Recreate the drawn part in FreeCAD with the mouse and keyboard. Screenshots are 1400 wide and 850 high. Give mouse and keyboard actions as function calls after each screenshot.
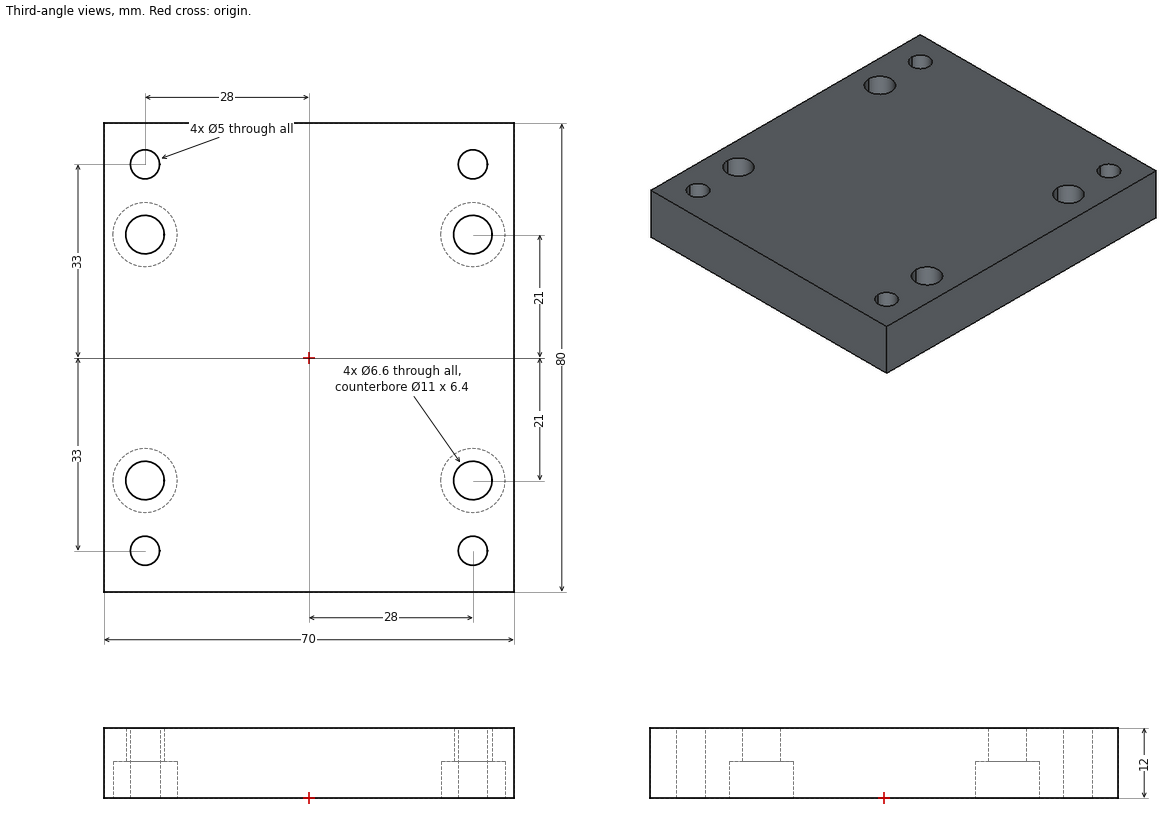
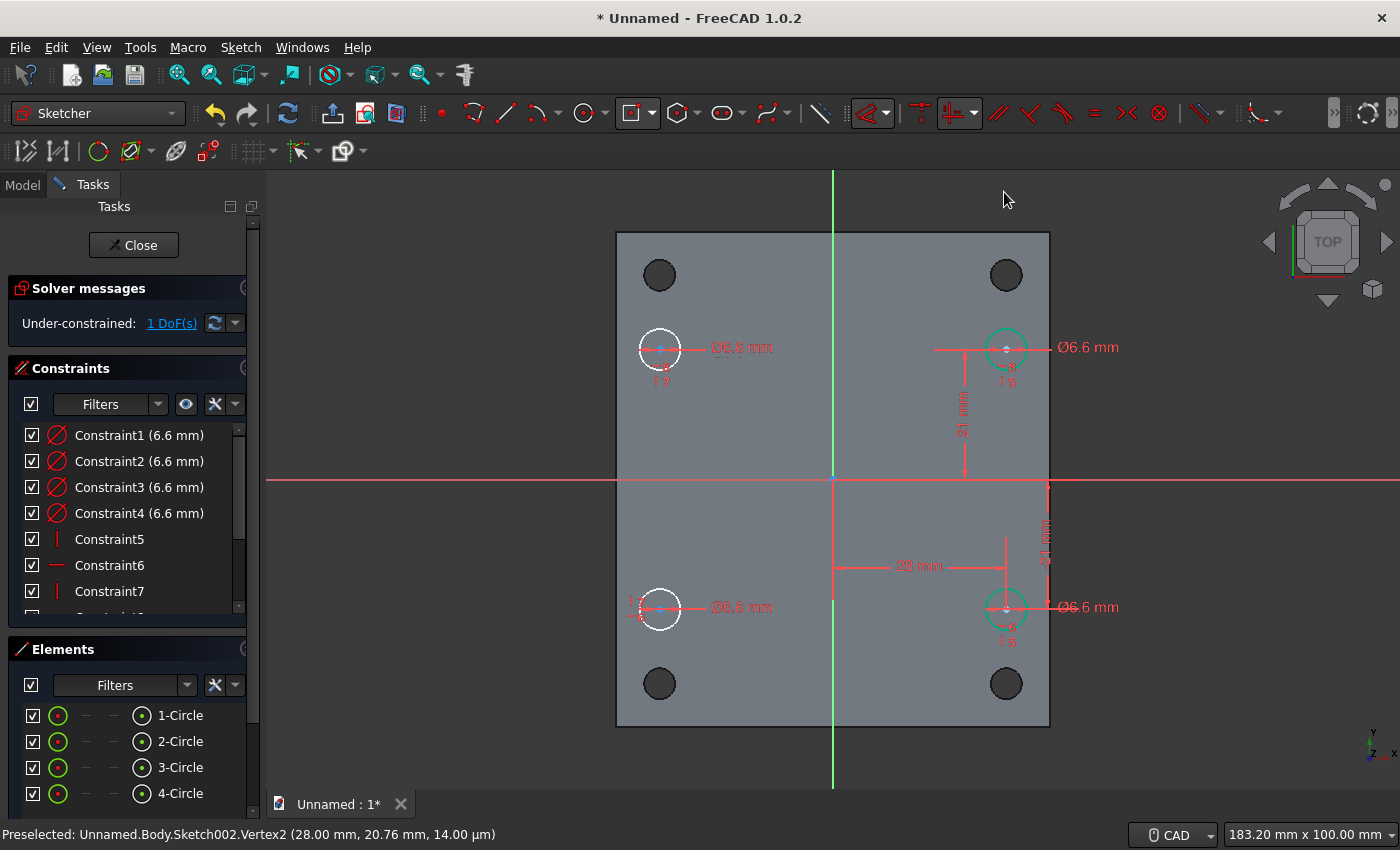
click(660, 609)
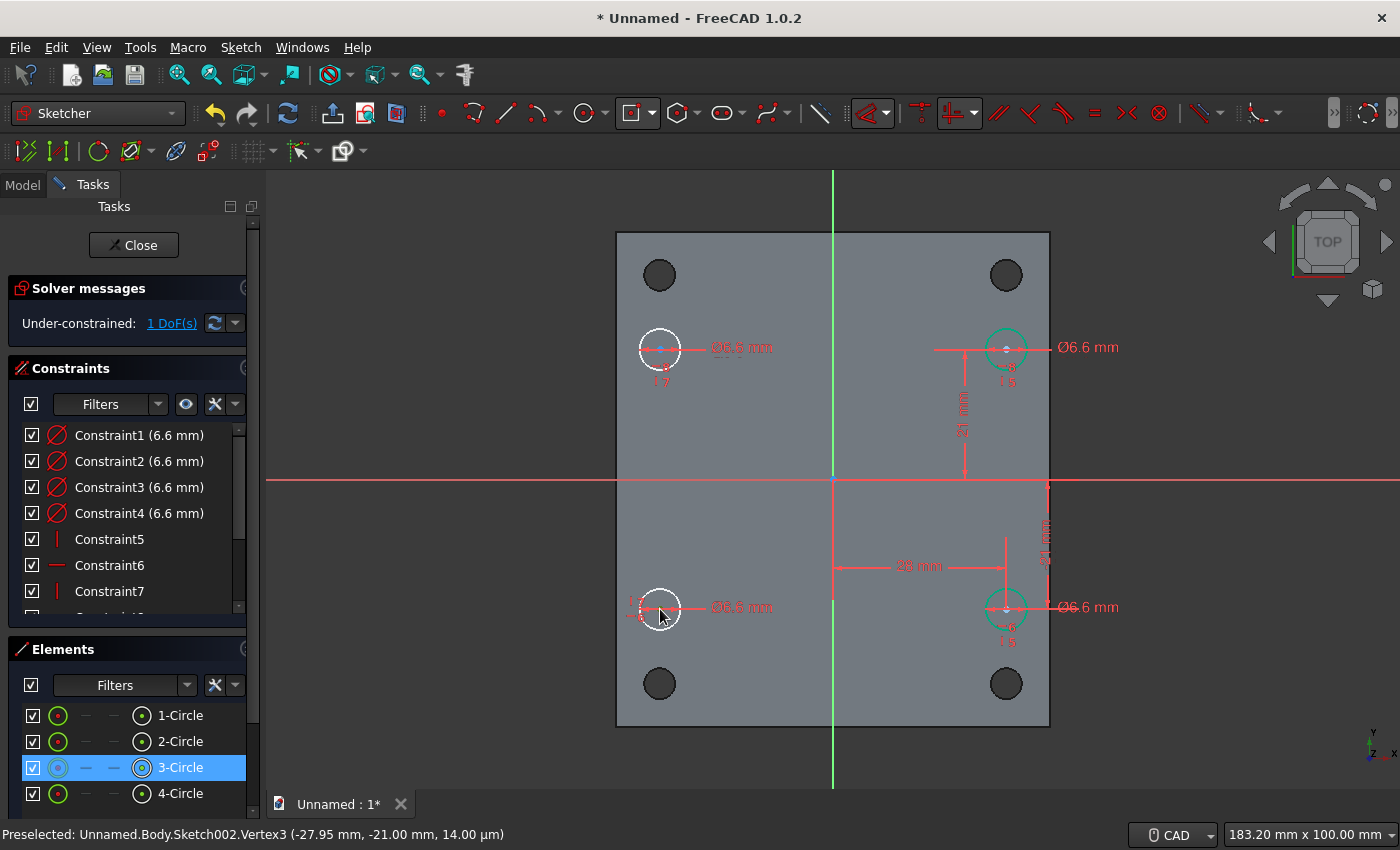
key(l)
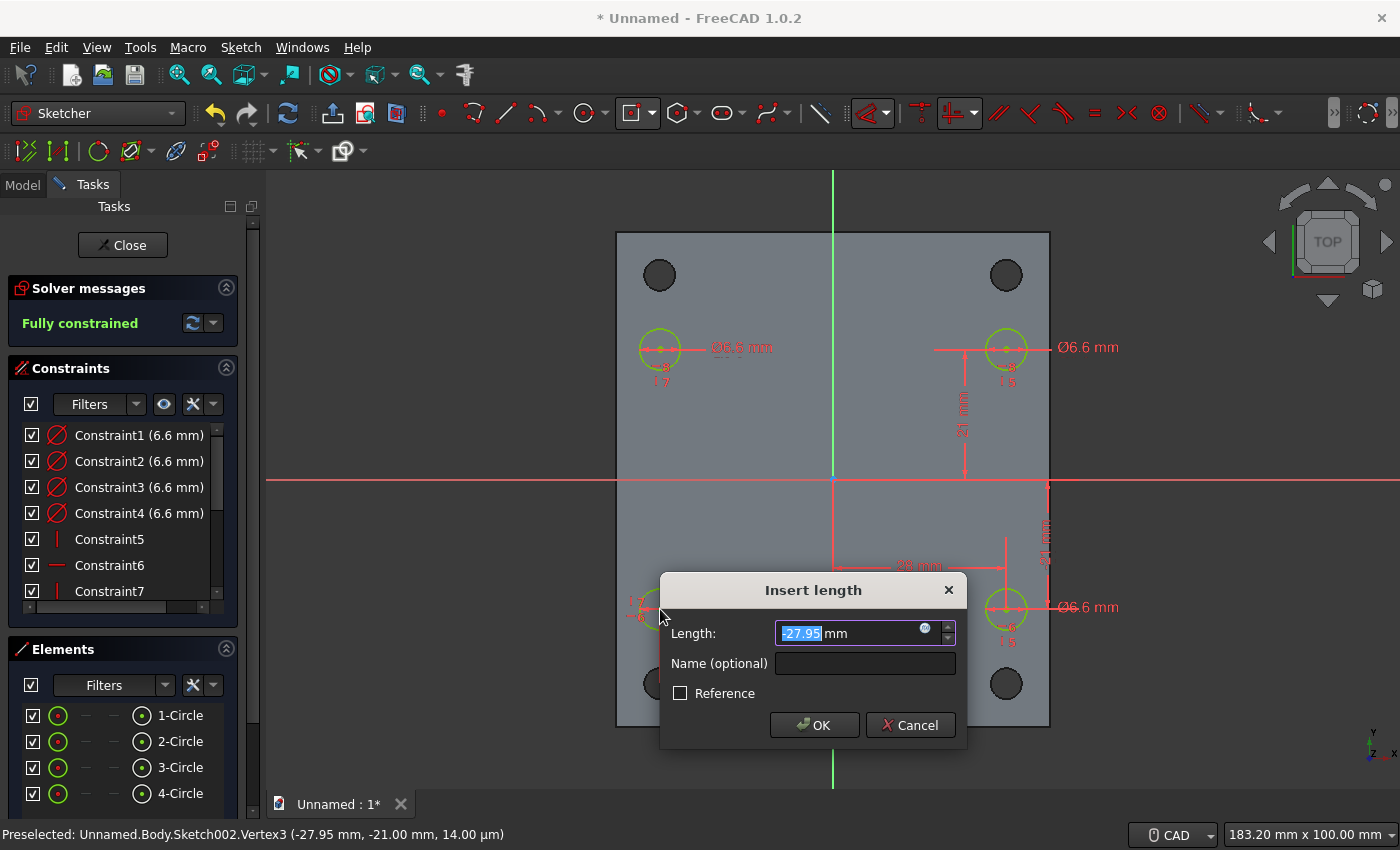
text(-28)
key(Return)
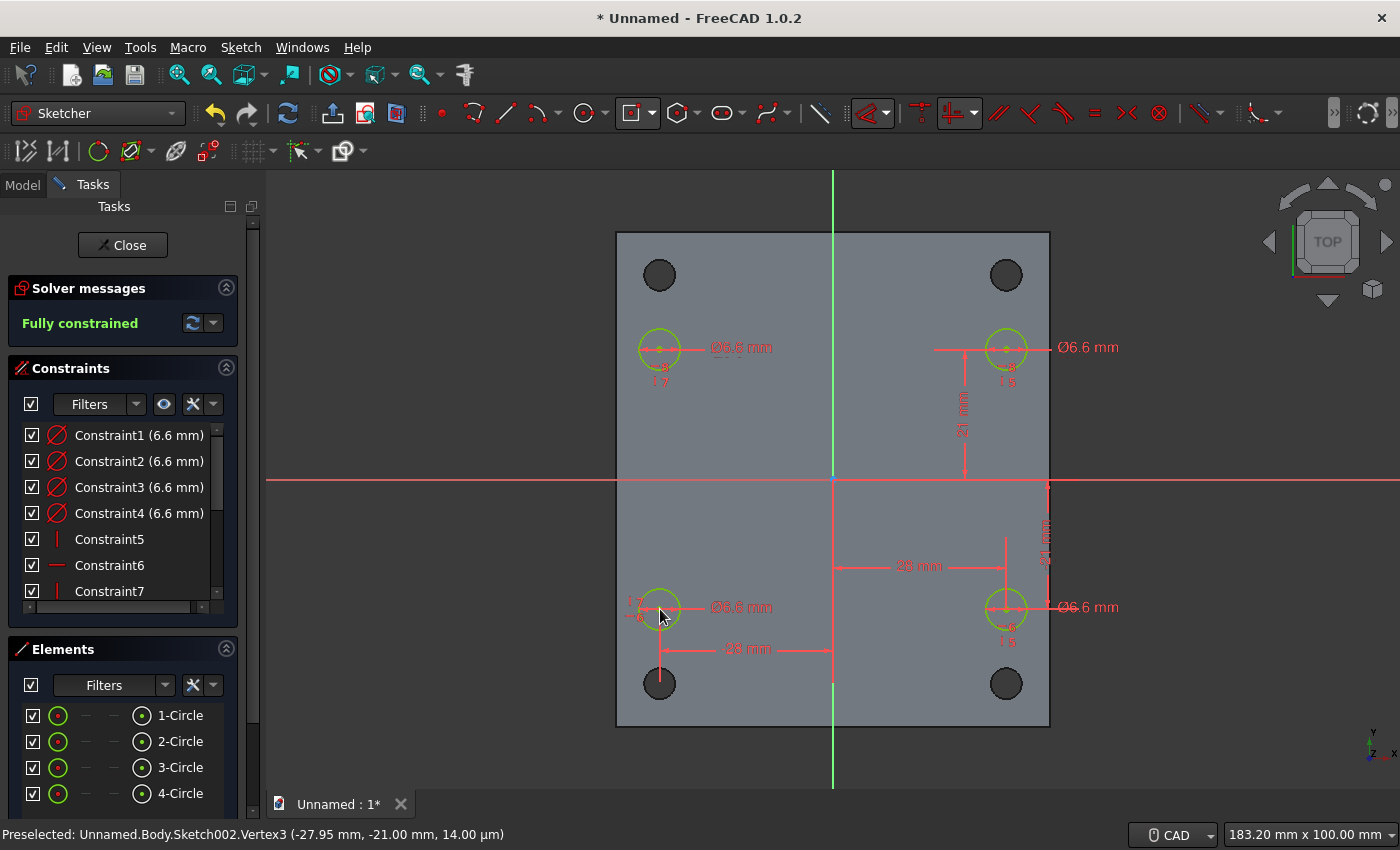
click(123, 245)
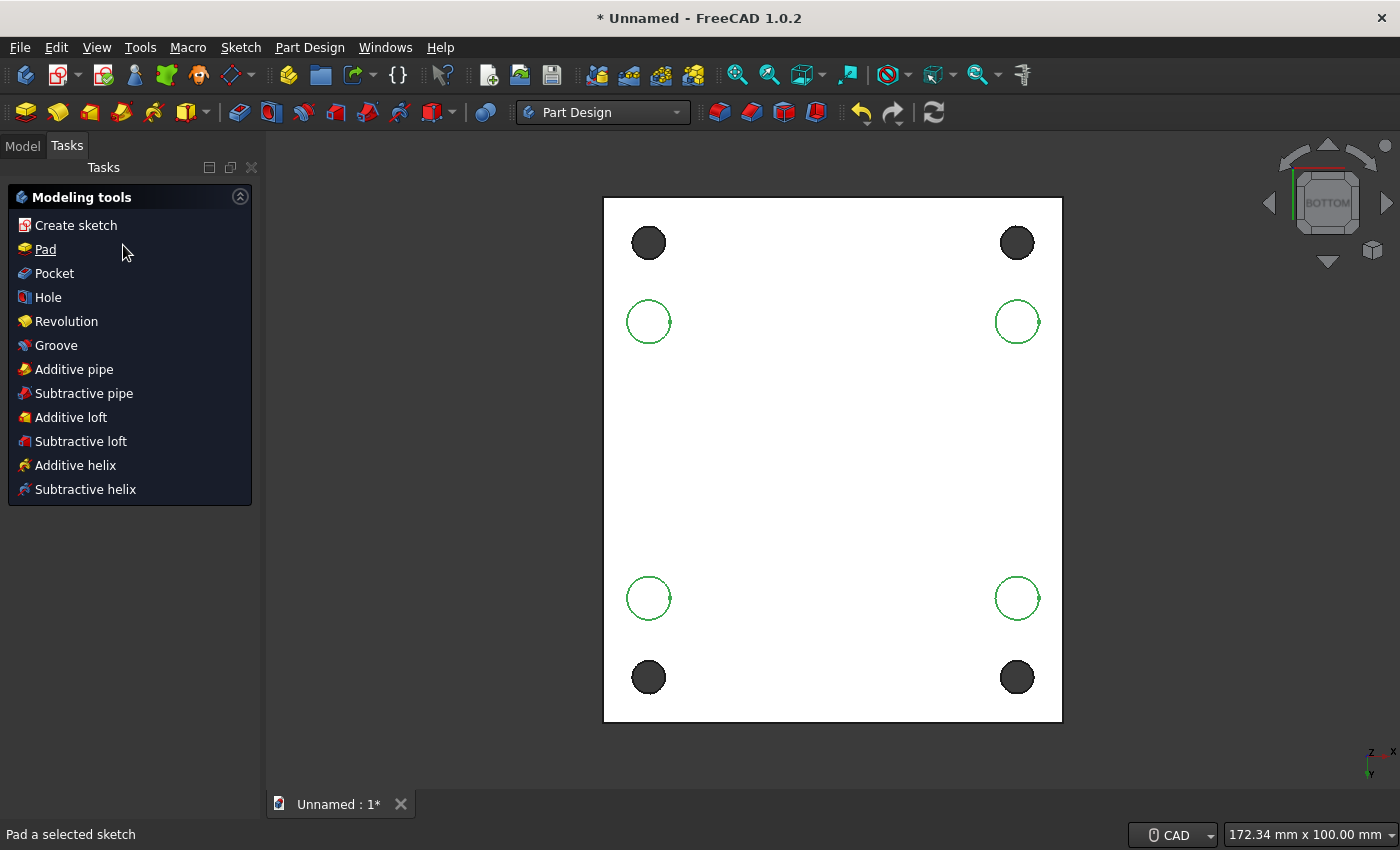
click(272, 112)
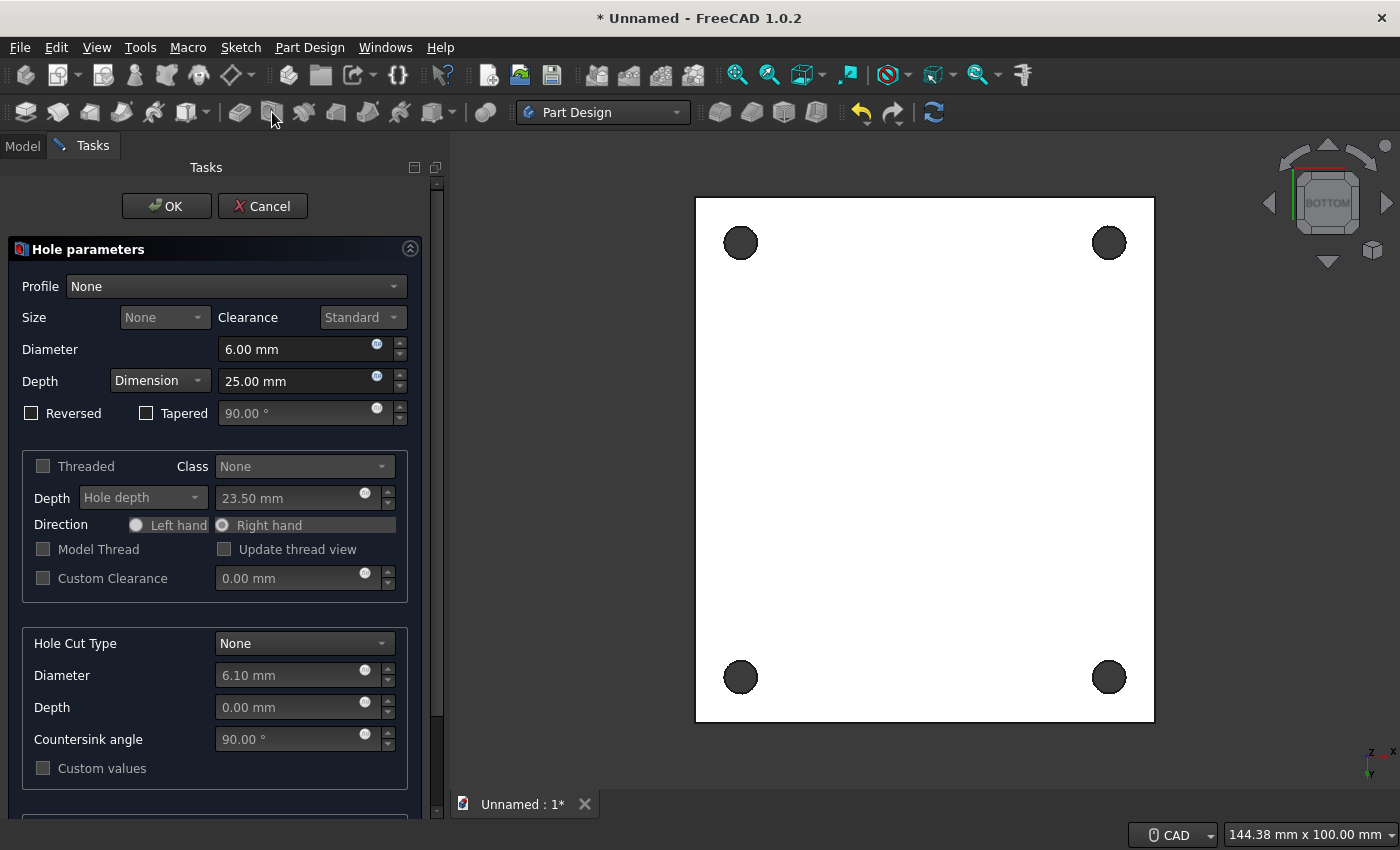
triple_click(305, 349)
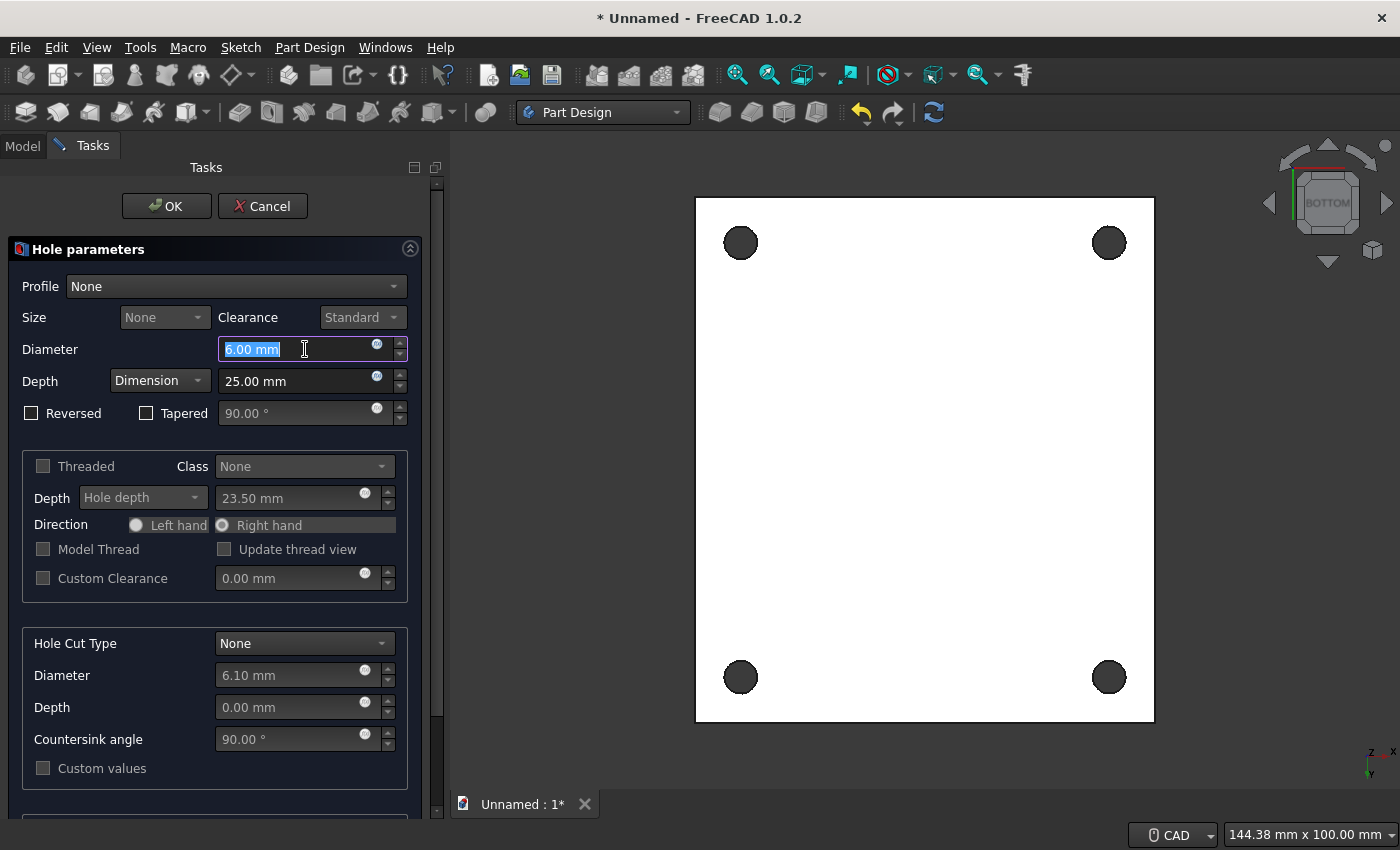
text(6.6)
key(Tab)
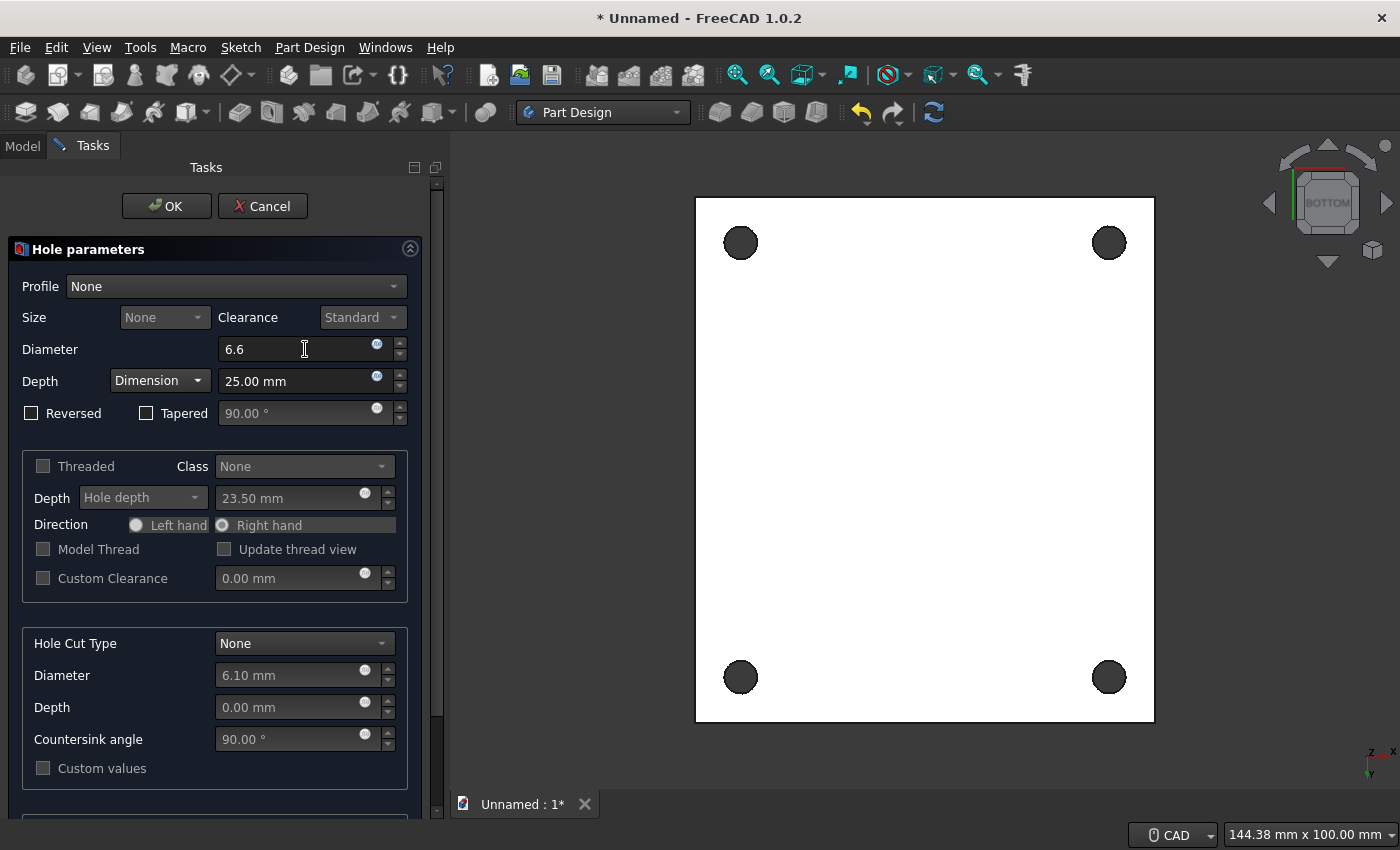
click(161, 380)